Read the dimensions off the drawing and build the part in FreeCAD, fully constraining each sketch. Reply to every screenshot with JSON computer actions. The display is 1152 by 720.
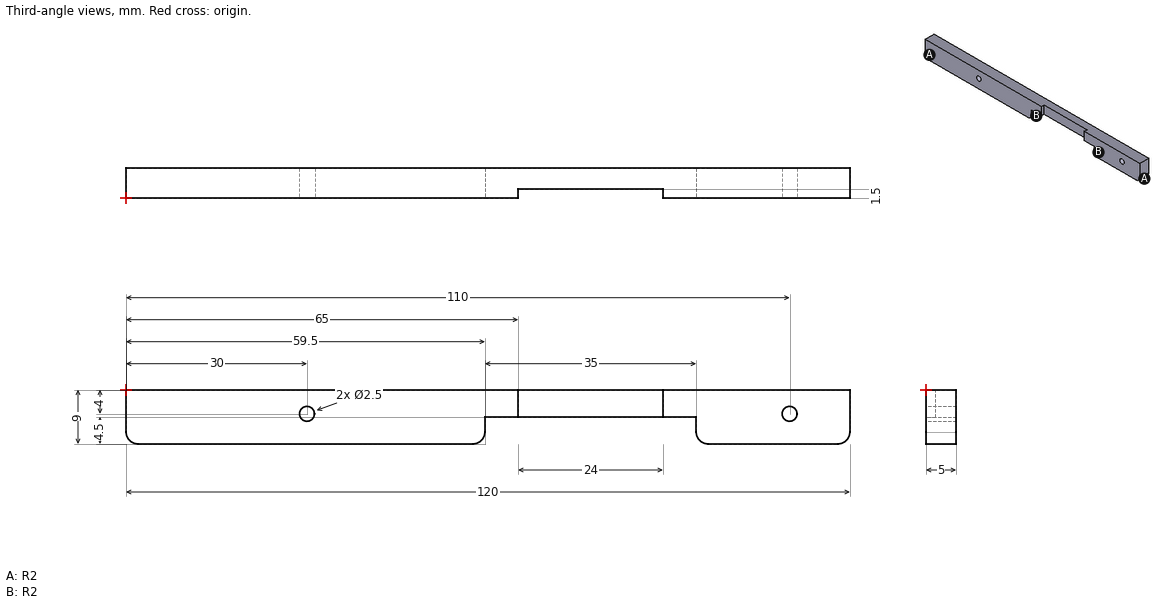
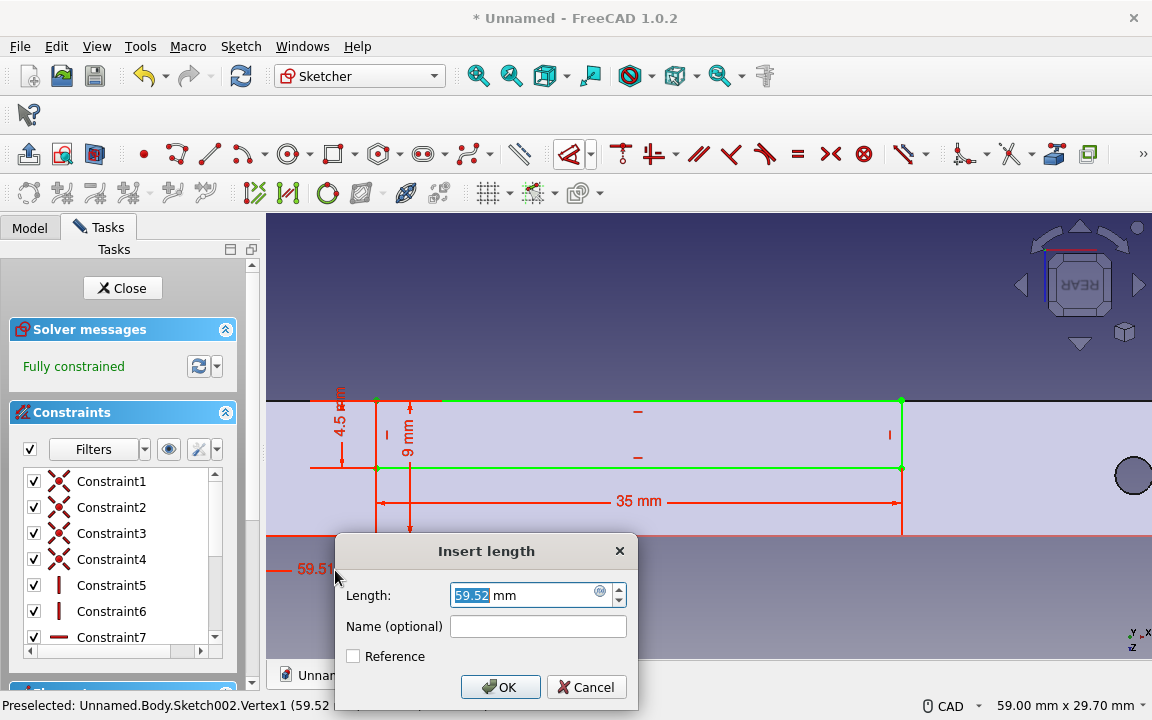
{"action": "type", "text": "59.5"}
{"action": "key", "text": "Return"}
{"action": "key", "text": "Escape"}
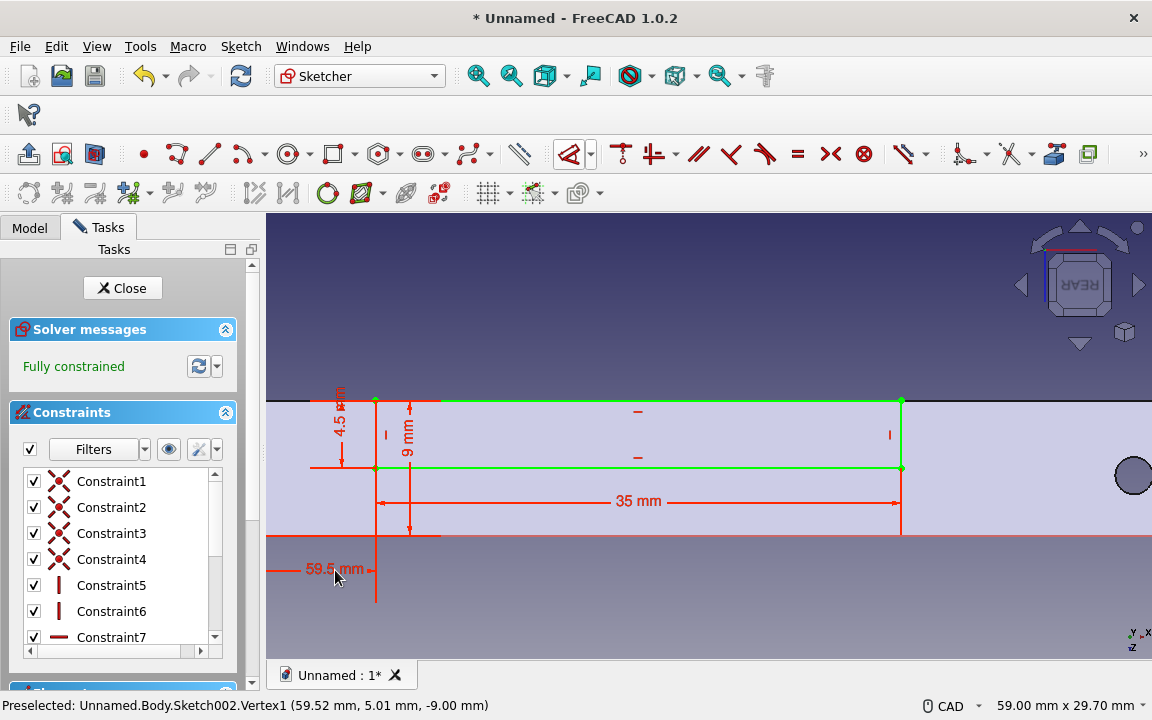
{"action": "left_click", "coordinate": [123, 288]}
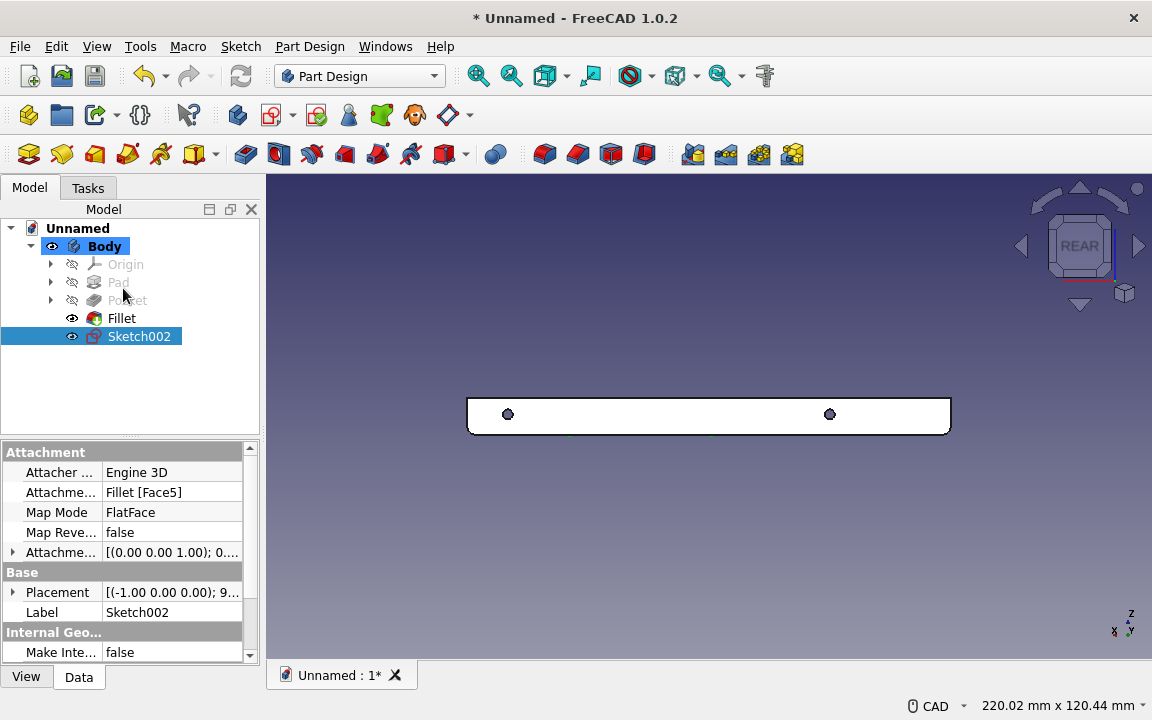
{"action": "left_click", "coordinate": [246, 154]}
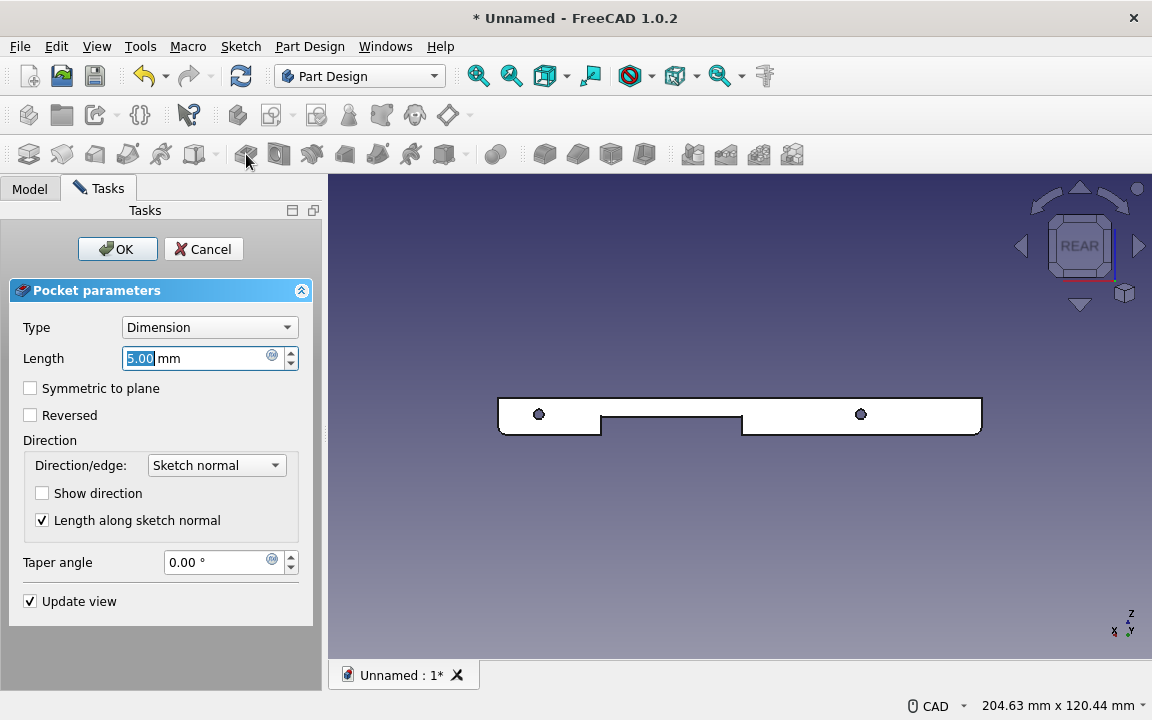
{"action": "left_click", "coordinate": [210, 328]}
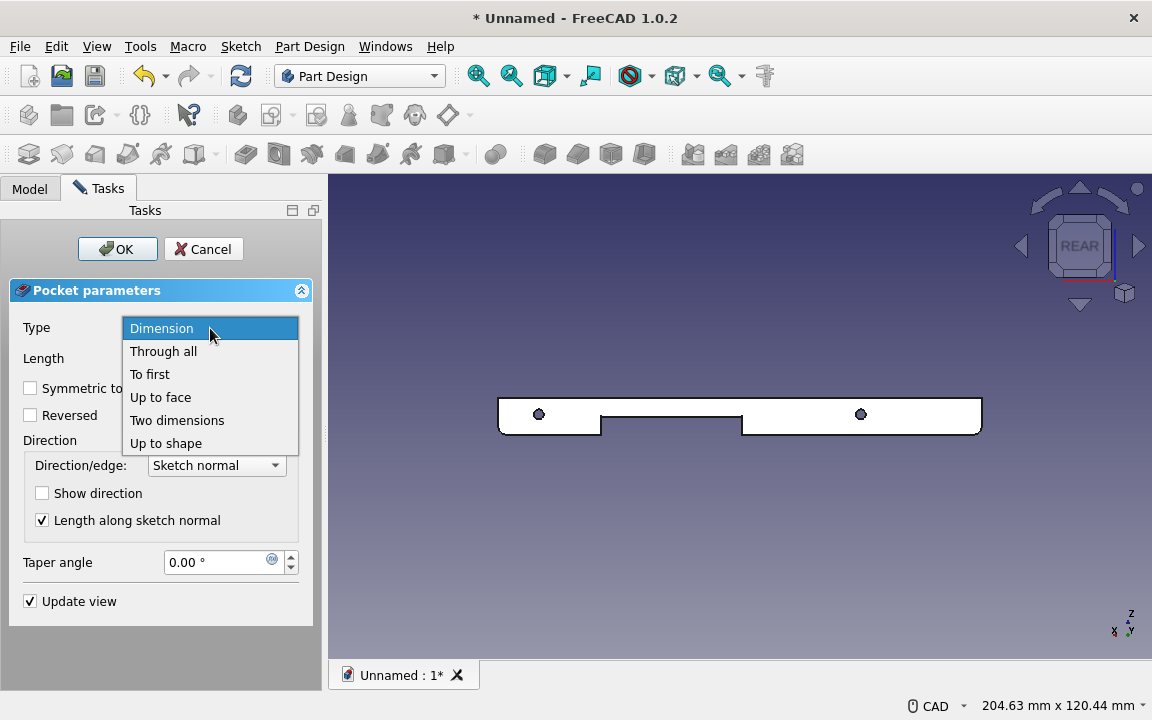
{"action": "left_click", "coordinate": [208, 352]}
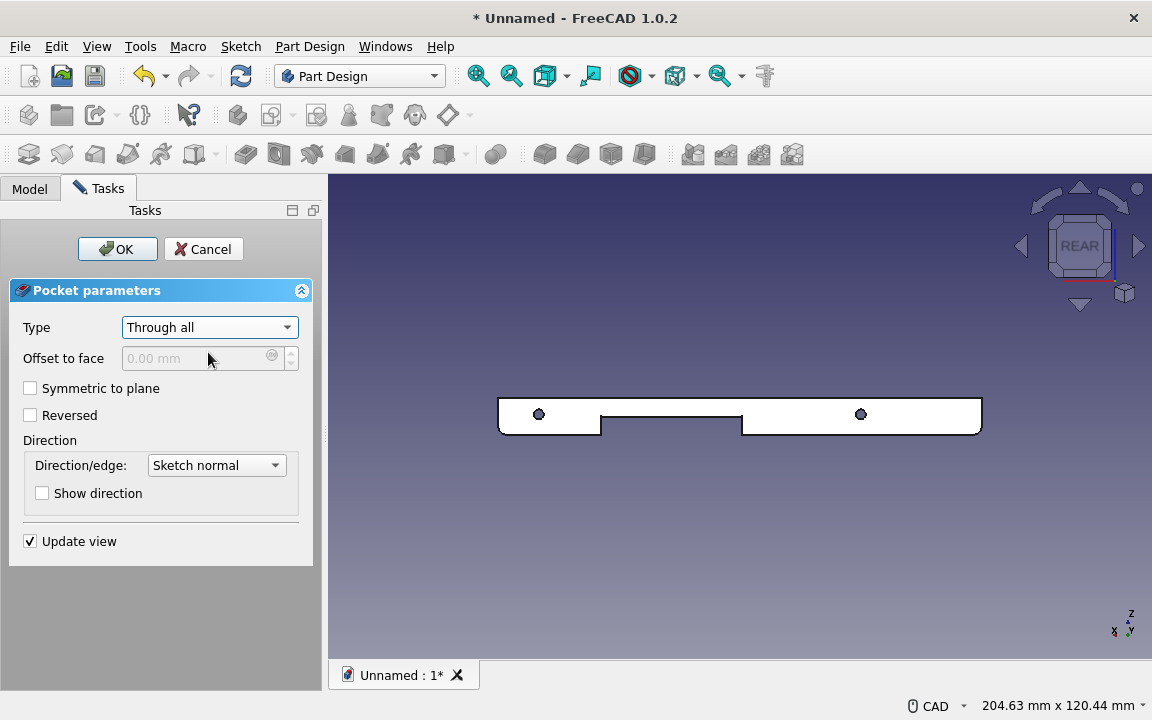
{"action": "left_click", "coordinate": [118, 249]}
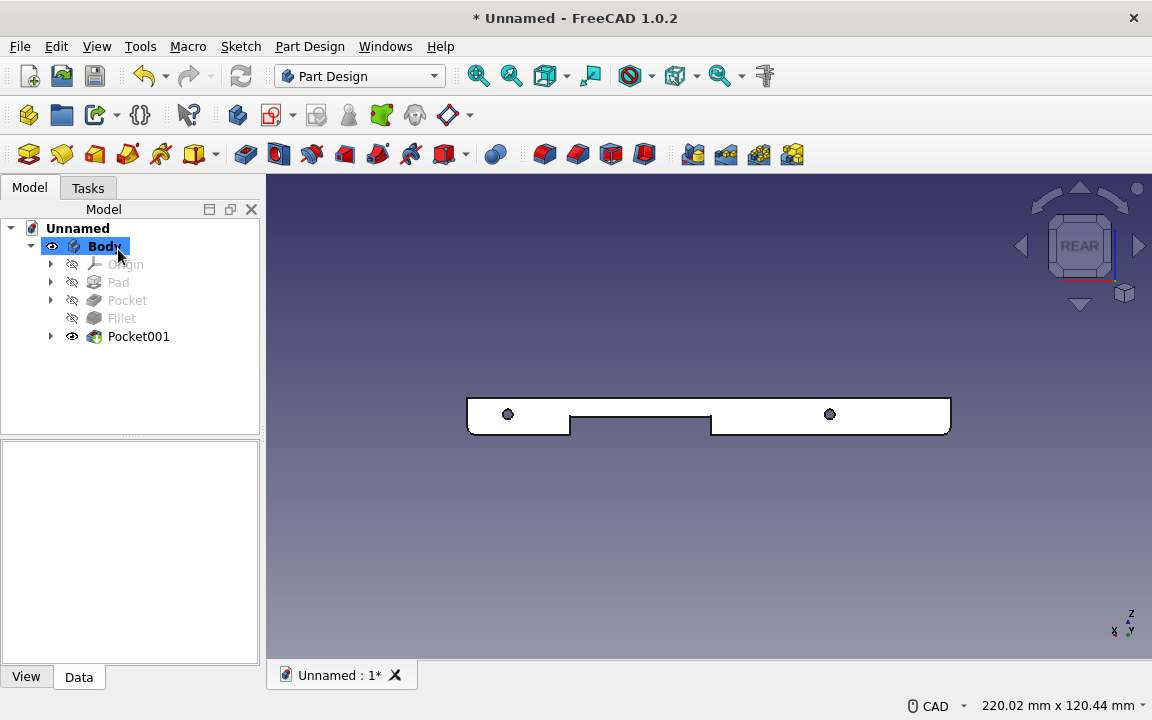
{"action": "scroll", "coordinate": [570, 434], "scroll_direction": "up", "scroll_amount": 4}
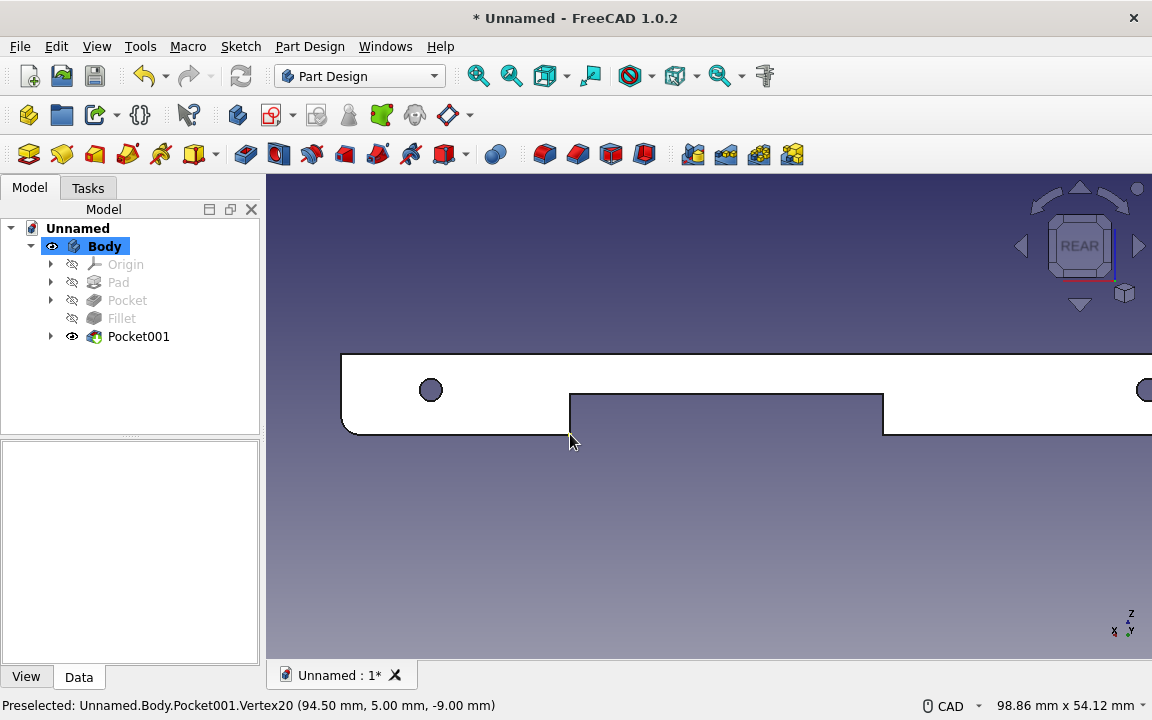
{"action": "key", "text": "v f"}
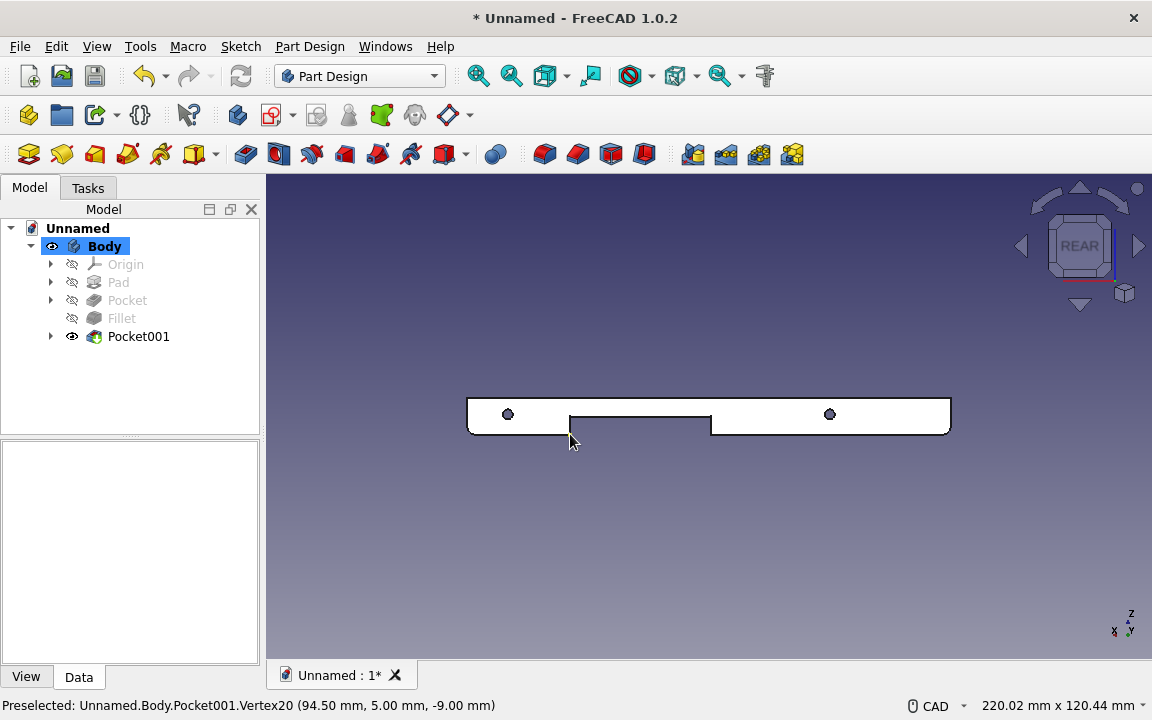
{"action": "key", "text": "0"}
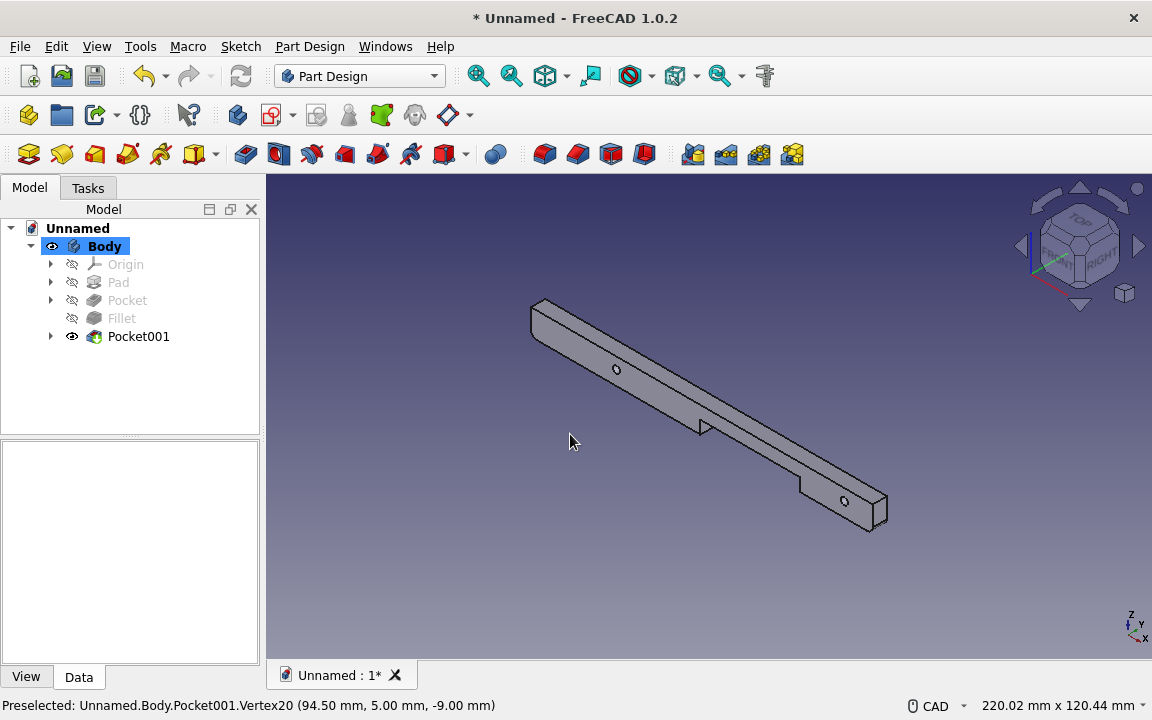
{"action": "scroll", "coordinate": [807, 487], "scroll_direction": "up", "scroll_amount": 4}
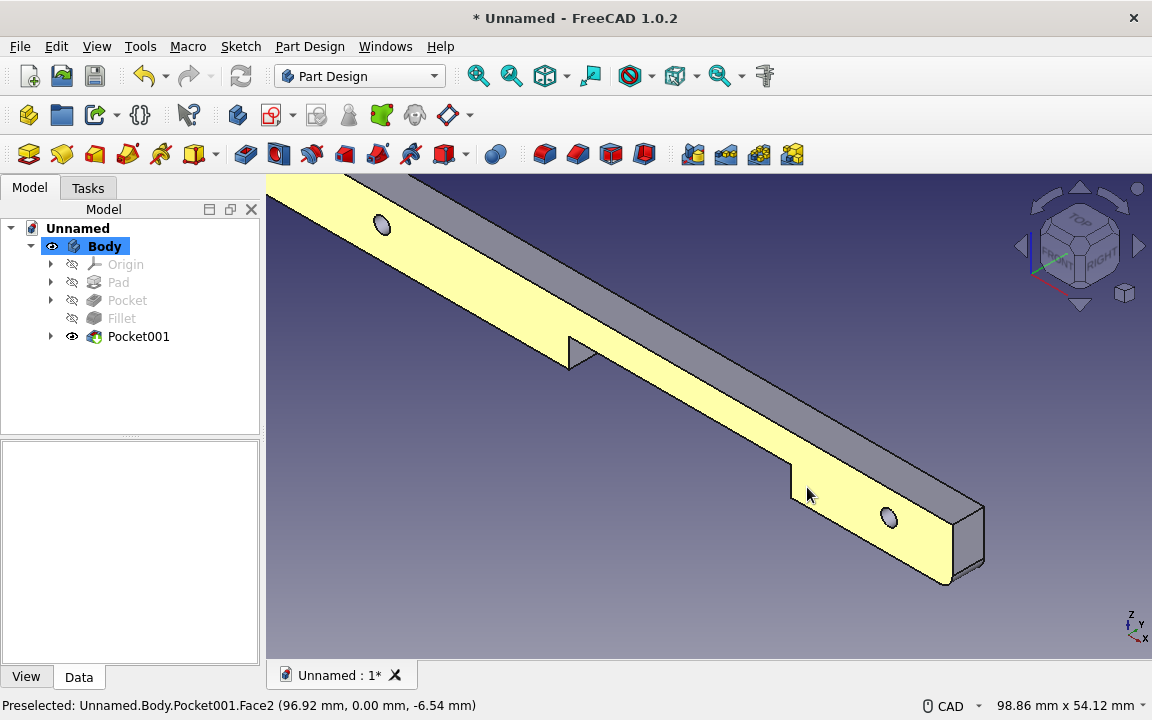
{"action": "key", "text": "v f"}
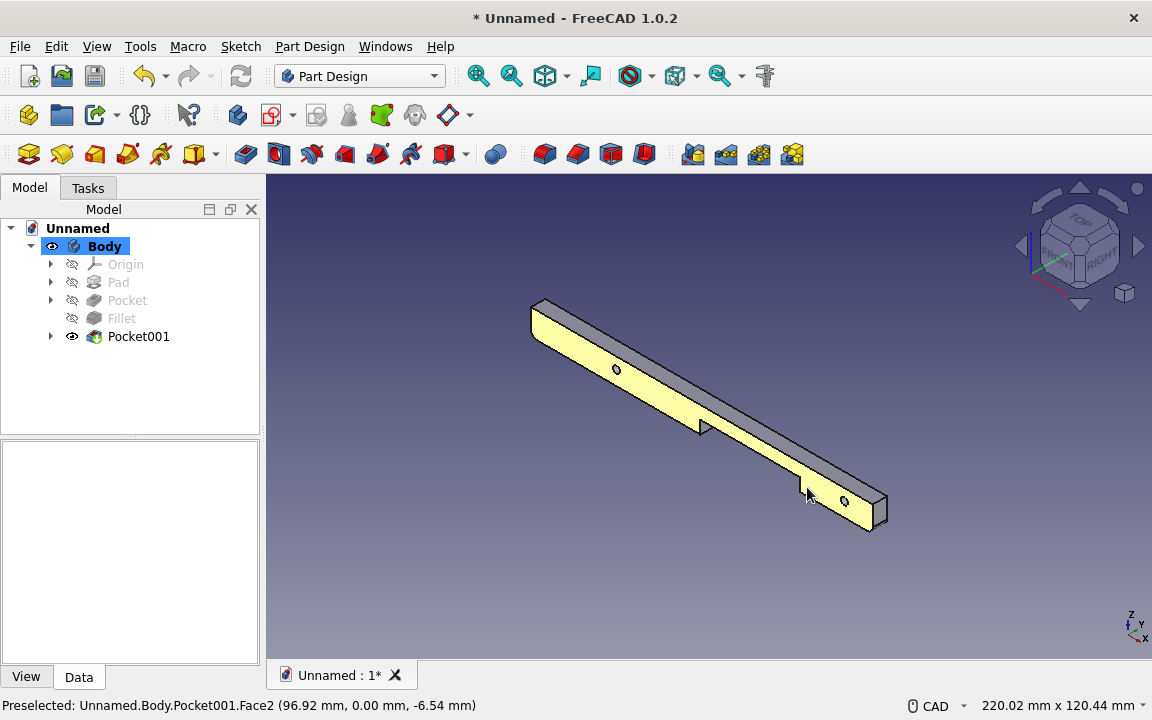
{"action": "key", "text": "2"}